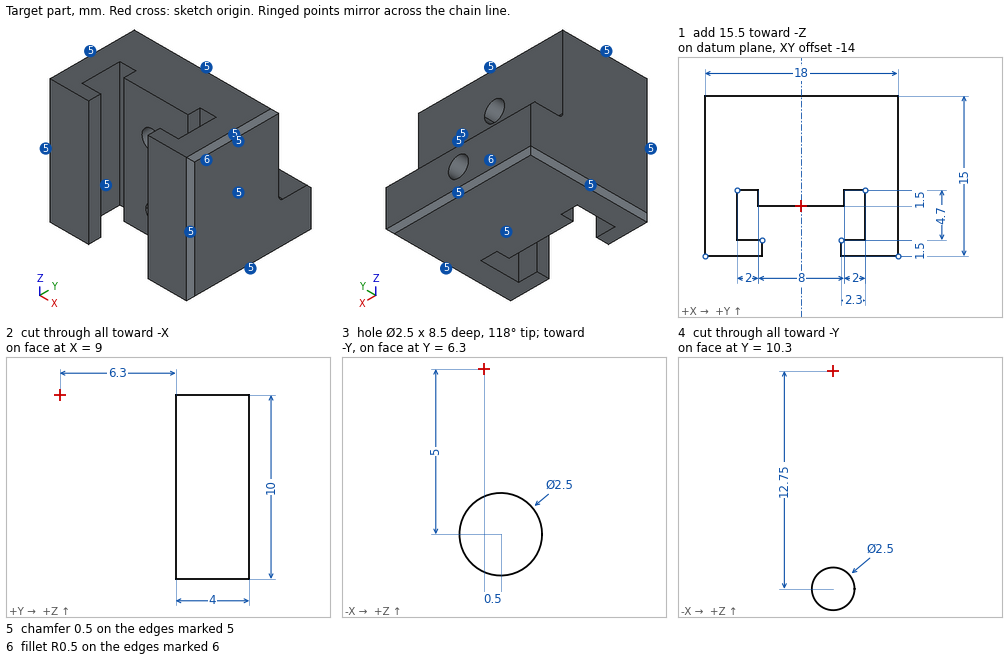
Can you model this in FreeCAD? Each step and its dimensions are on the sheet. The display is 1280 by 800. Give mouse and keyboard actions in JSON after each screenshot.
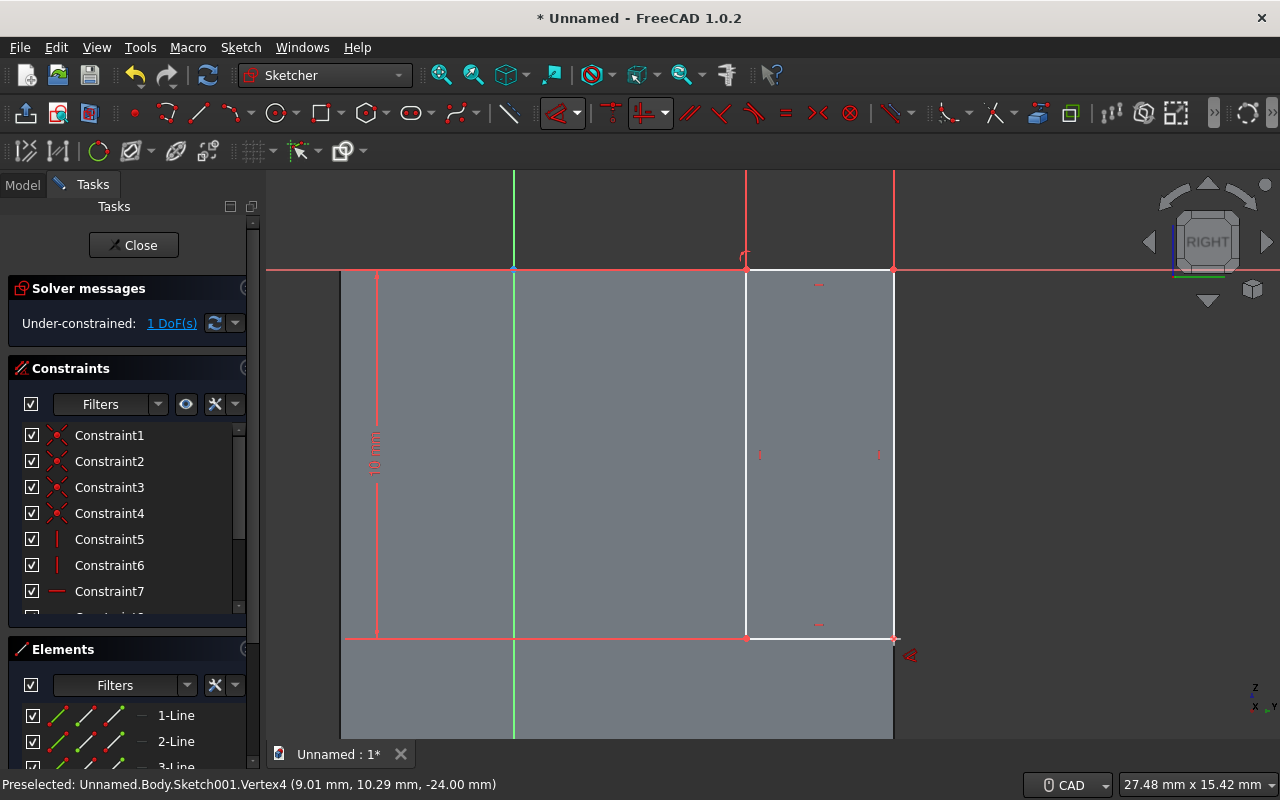
{"action": "left_click", "coordinate": [746, 270]}
{"action": "left_click", "coordinate": [630, 236]}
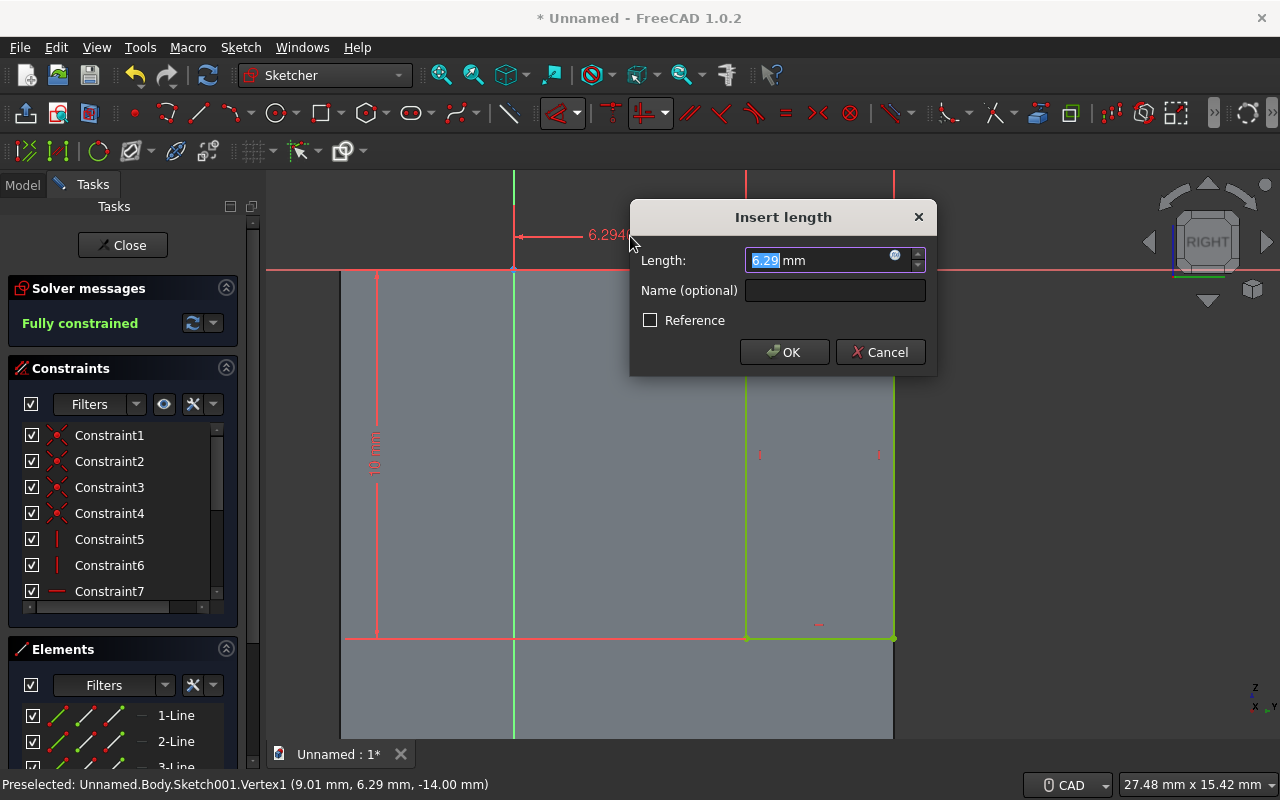
{"action": "type", "text": "6.3"}
{"action": "key", "text": "Return"}
{"action": "key", "text": "Escape"}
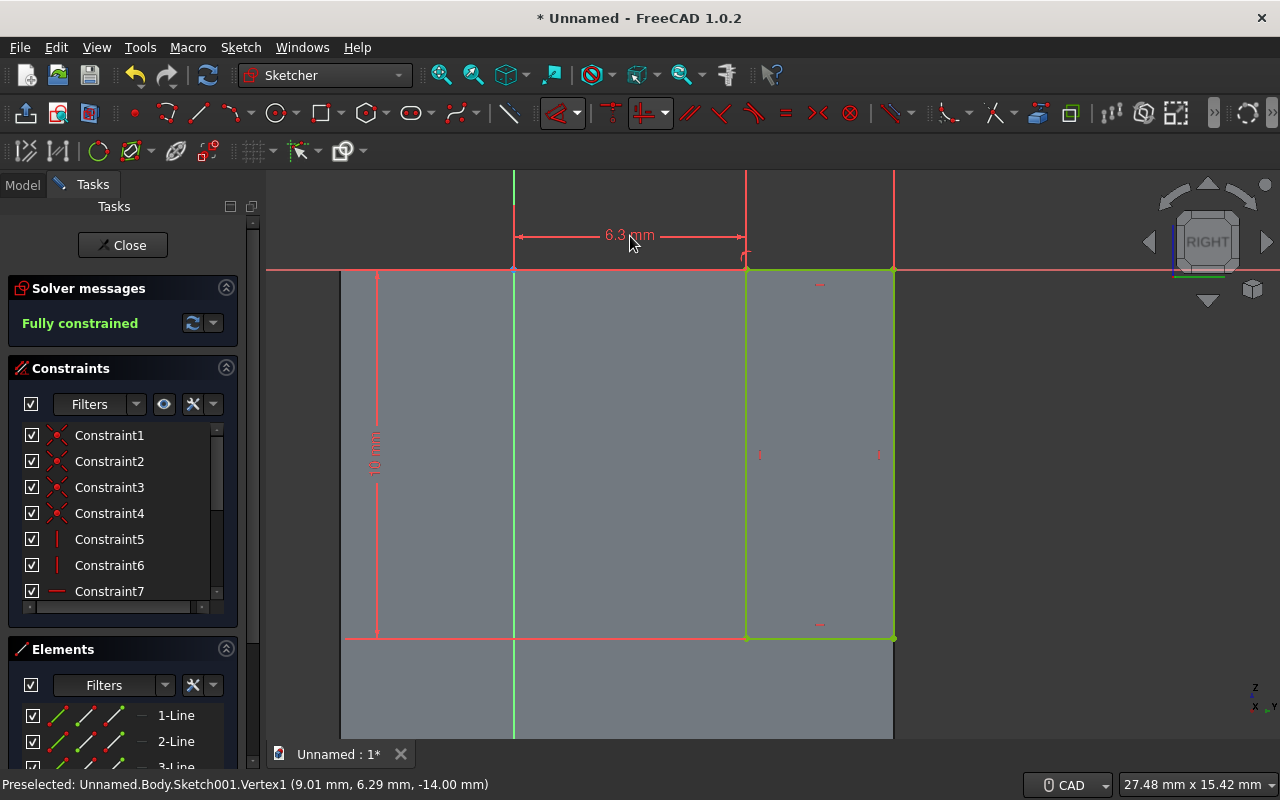
{"action": "left_click", "coordinate": [123, 245]}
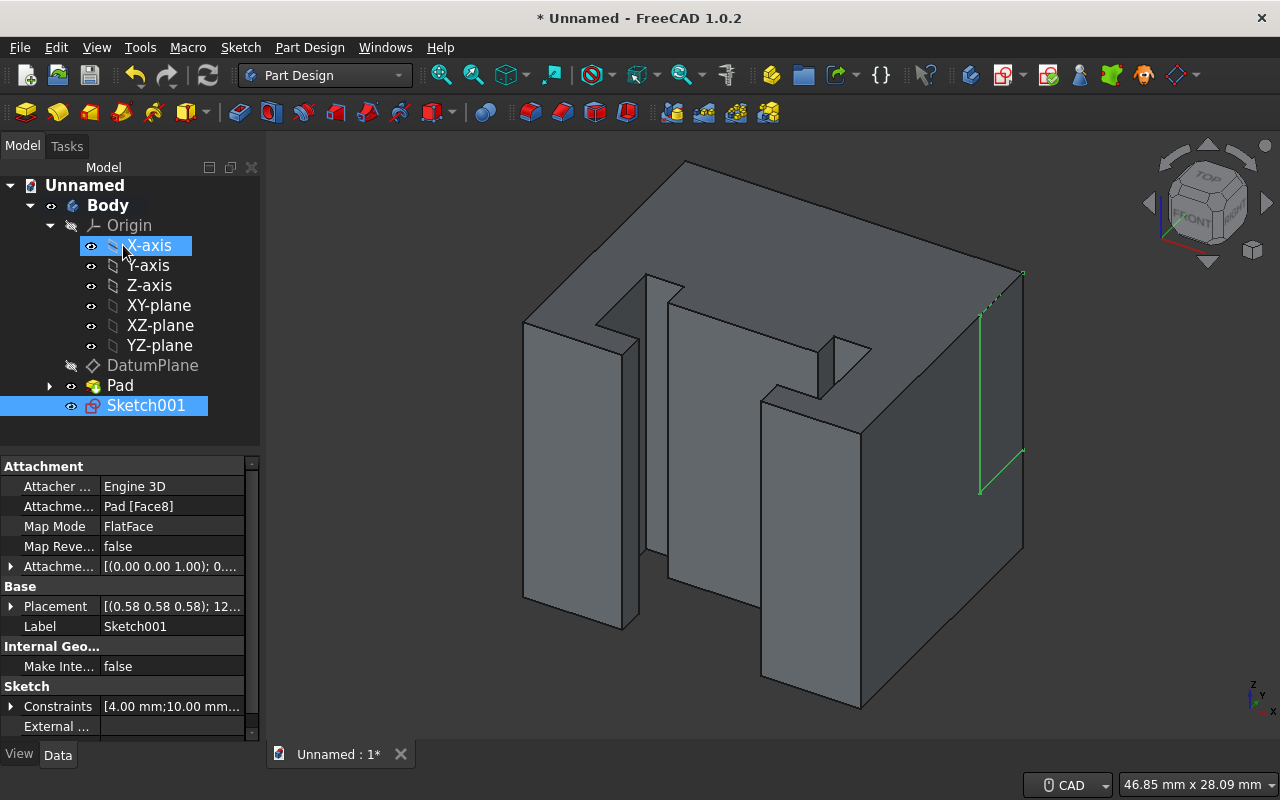
{"action": "left_click", "coordinate": [240, 112]}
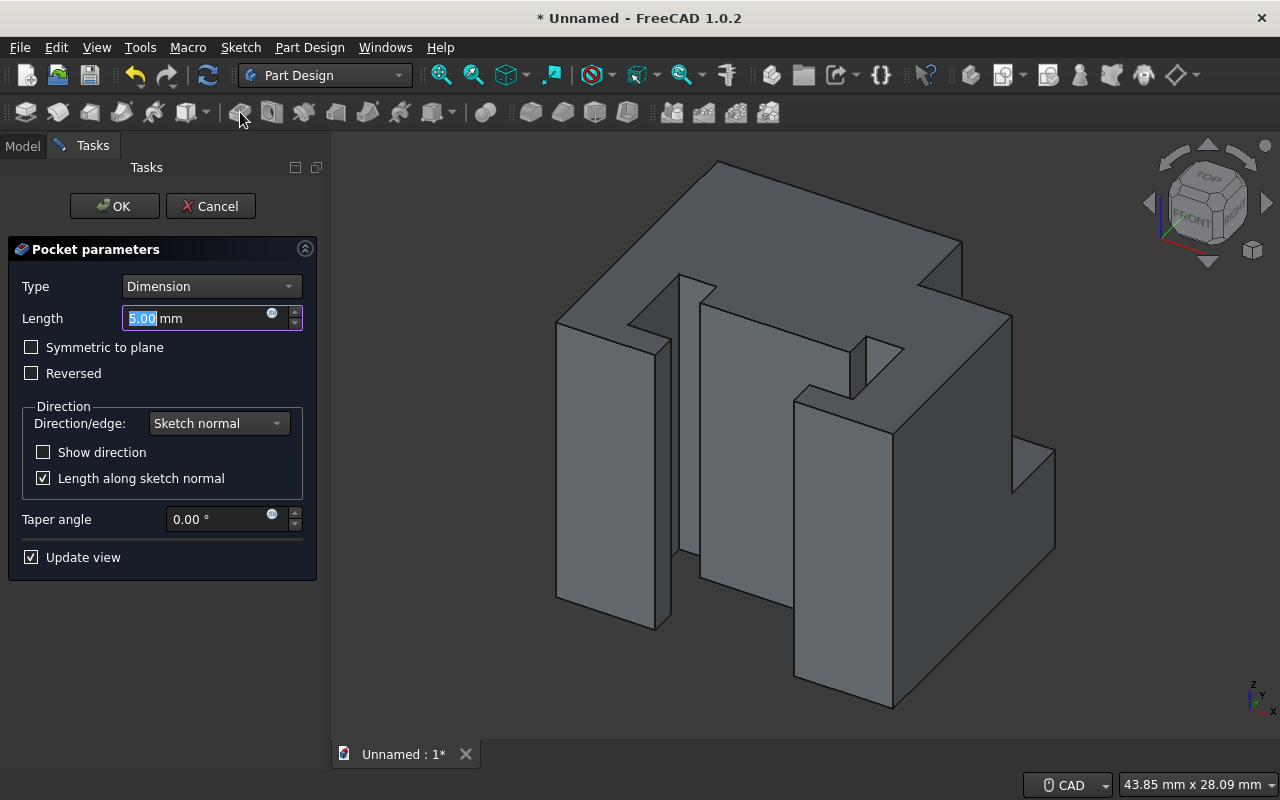
{"action": "left_click", "coordinate": [212, 286]}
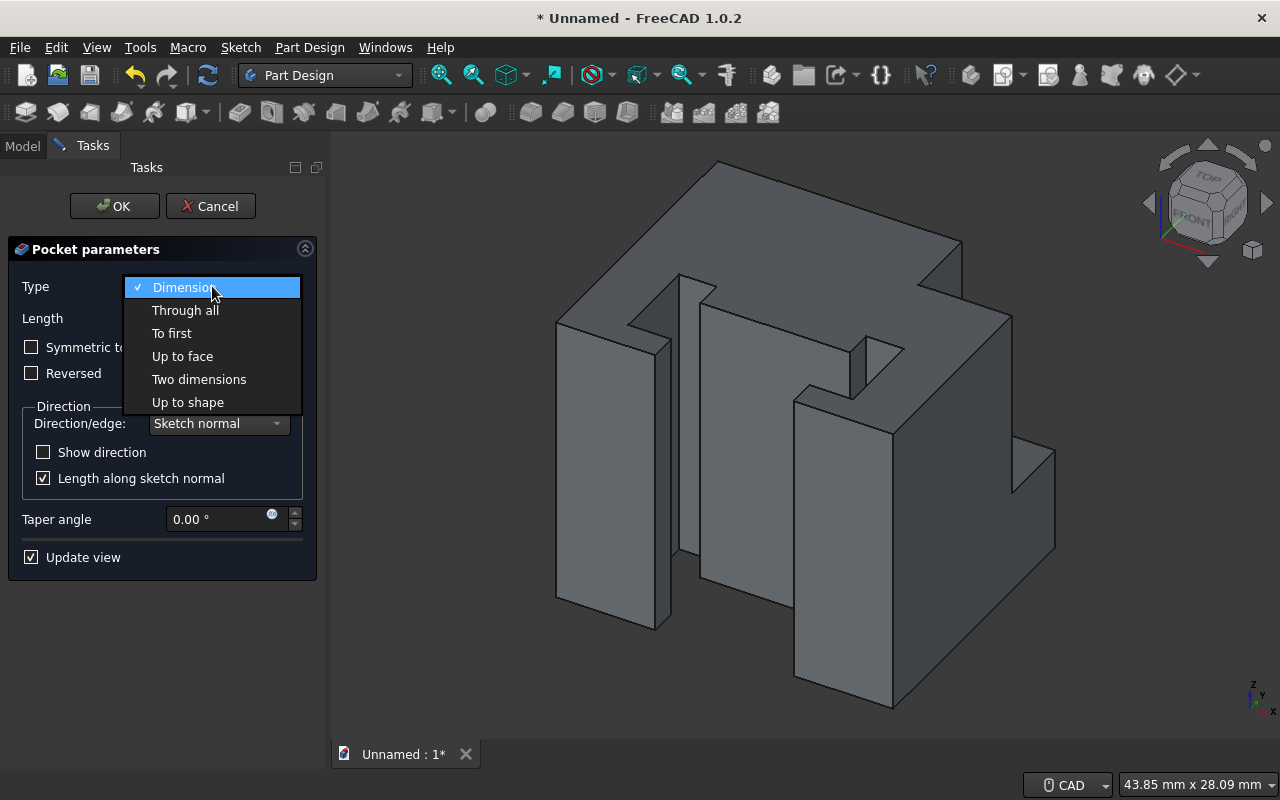
{"action": "left_click", "coordinate": [212, 310]}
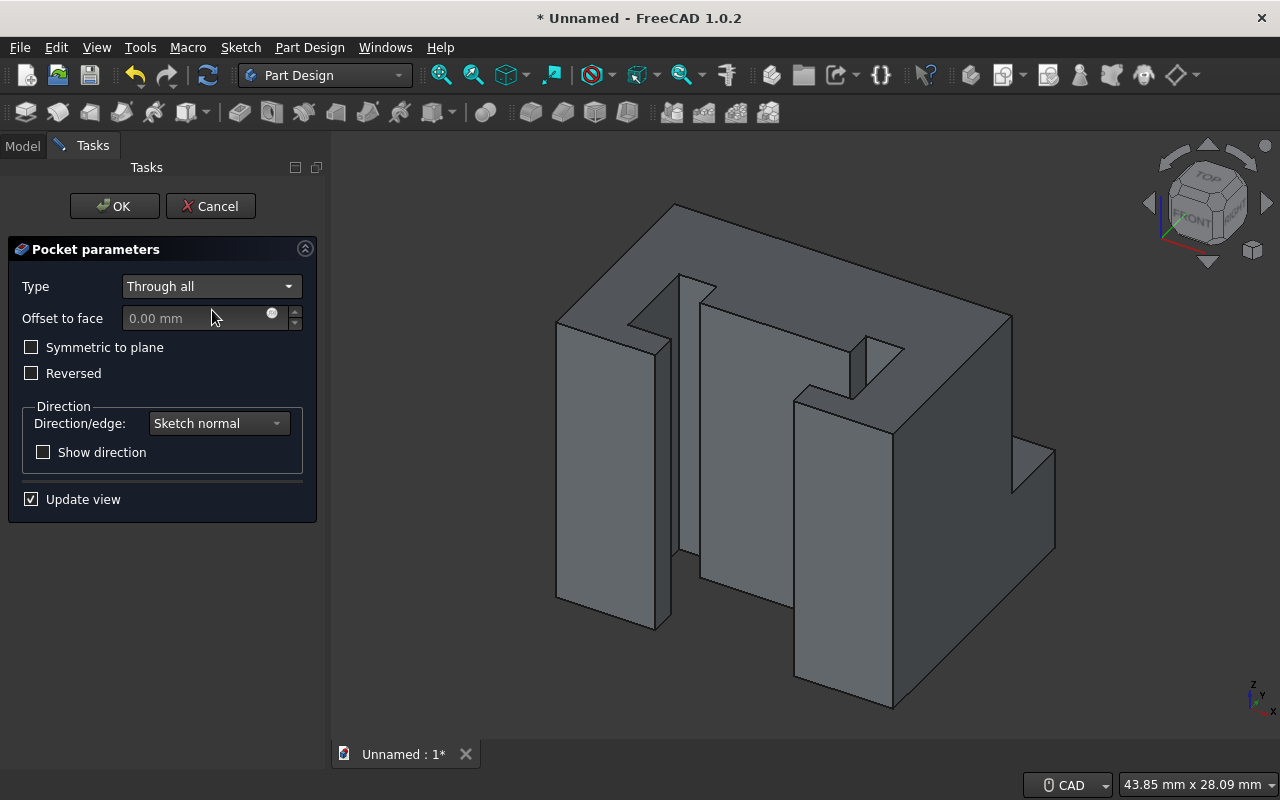
{"action": "left_click", "coordinate": [115, 206]}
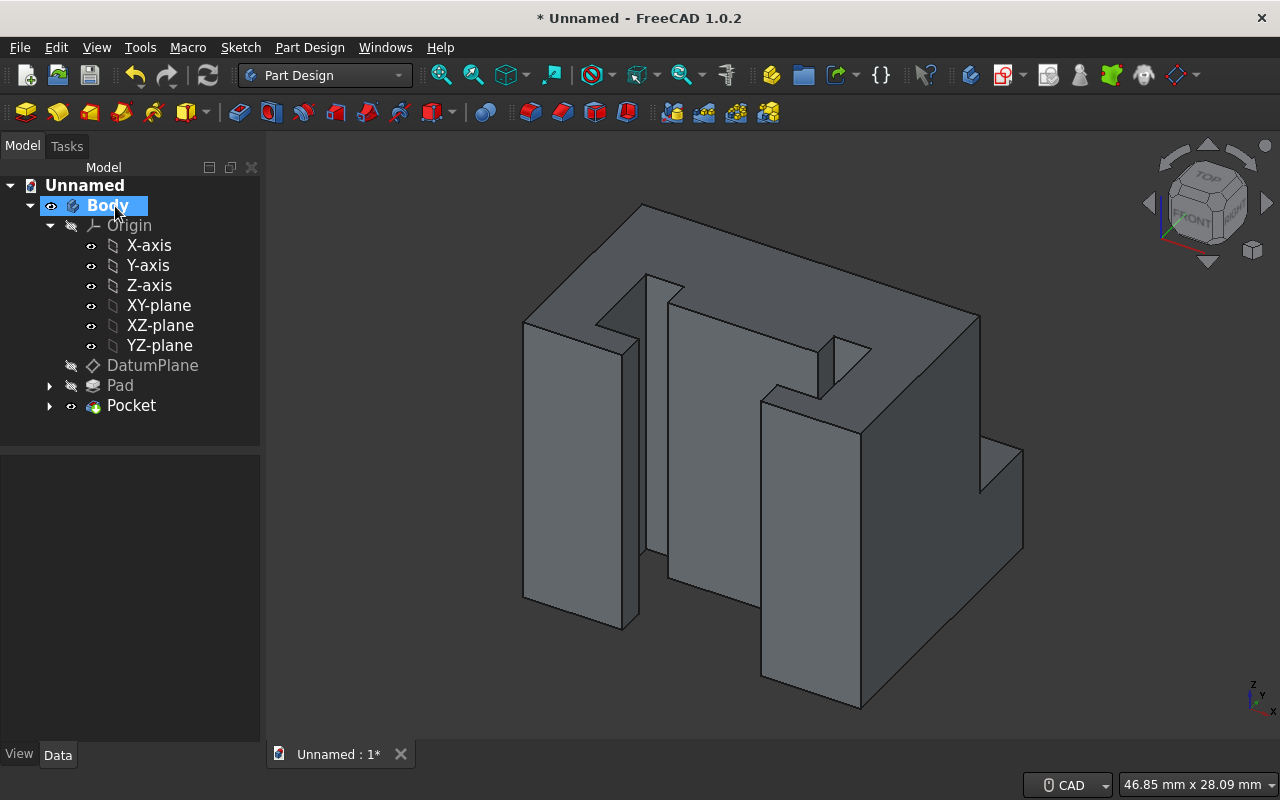
{"action": "key", "text": "4"}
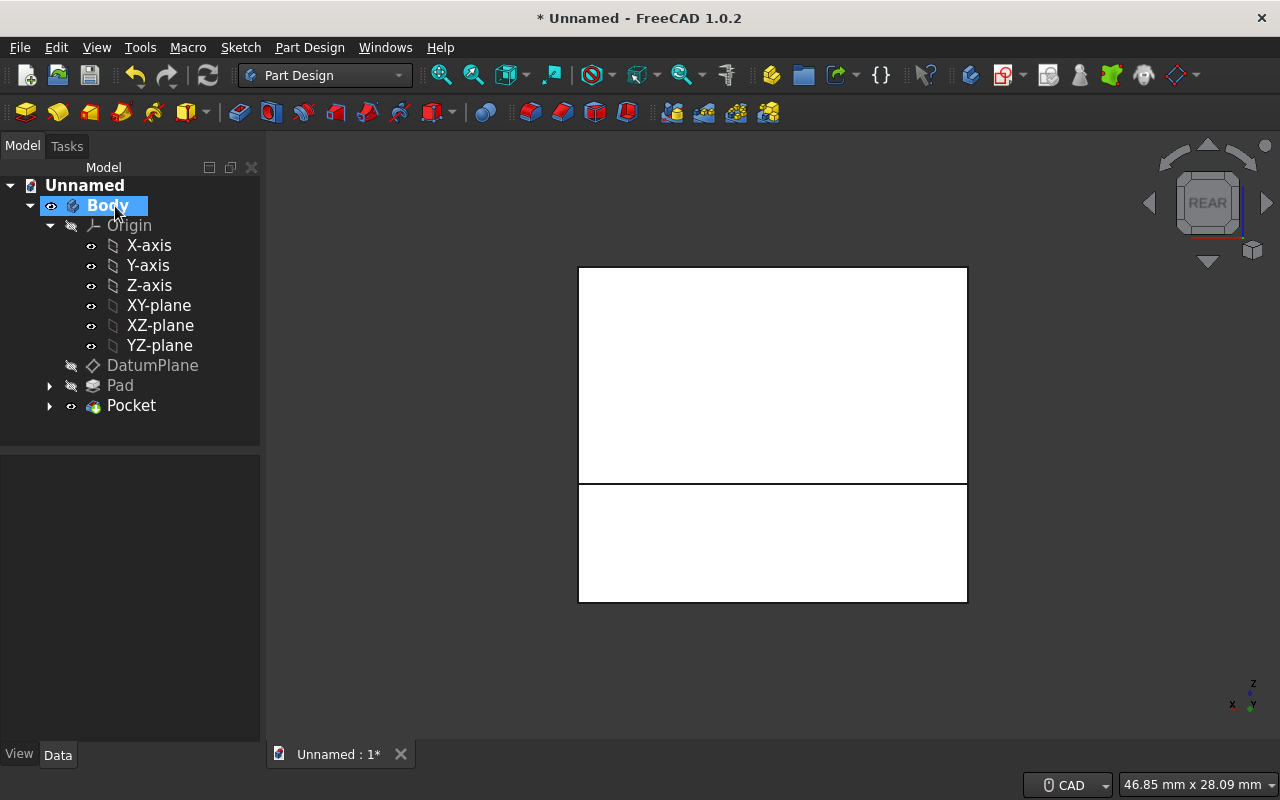
{"action": "left_click", "coordinate": [717, 374]}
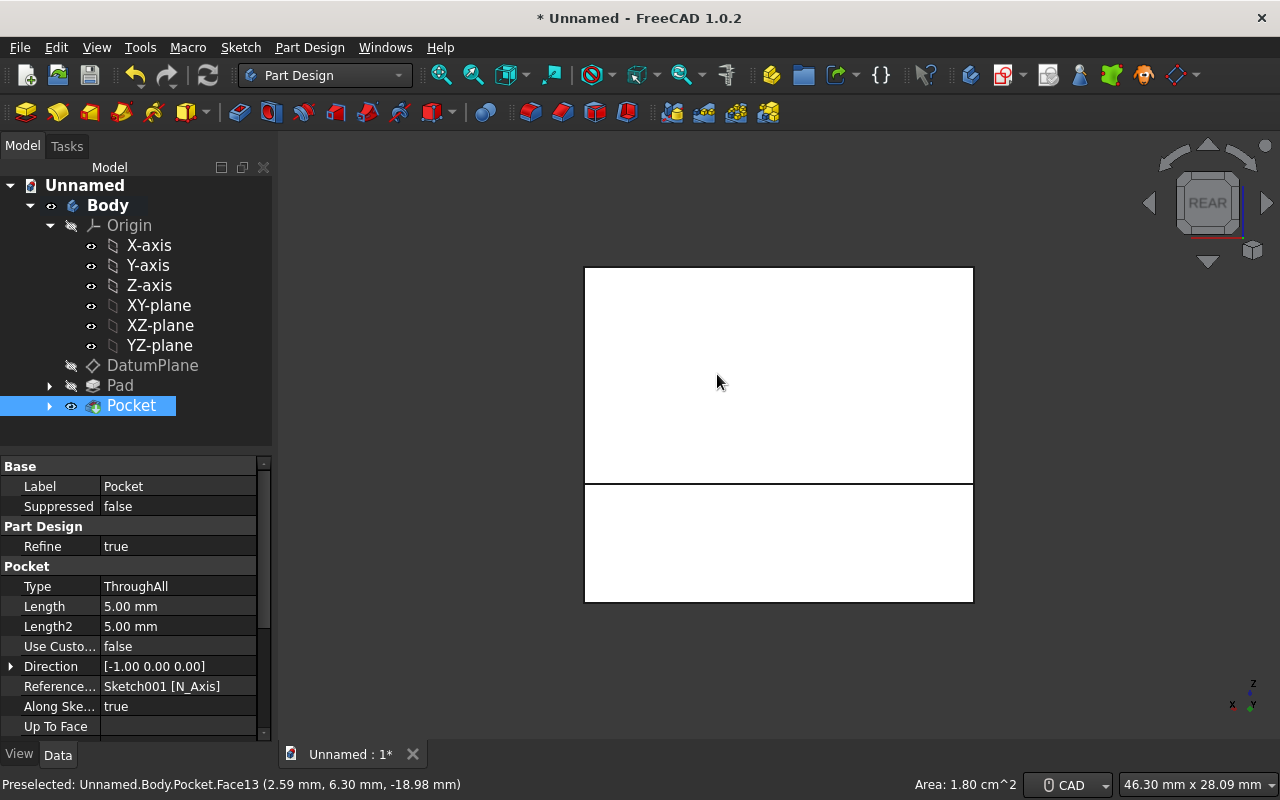
{"action": "left_click", "coordinate": [1004, 76]}